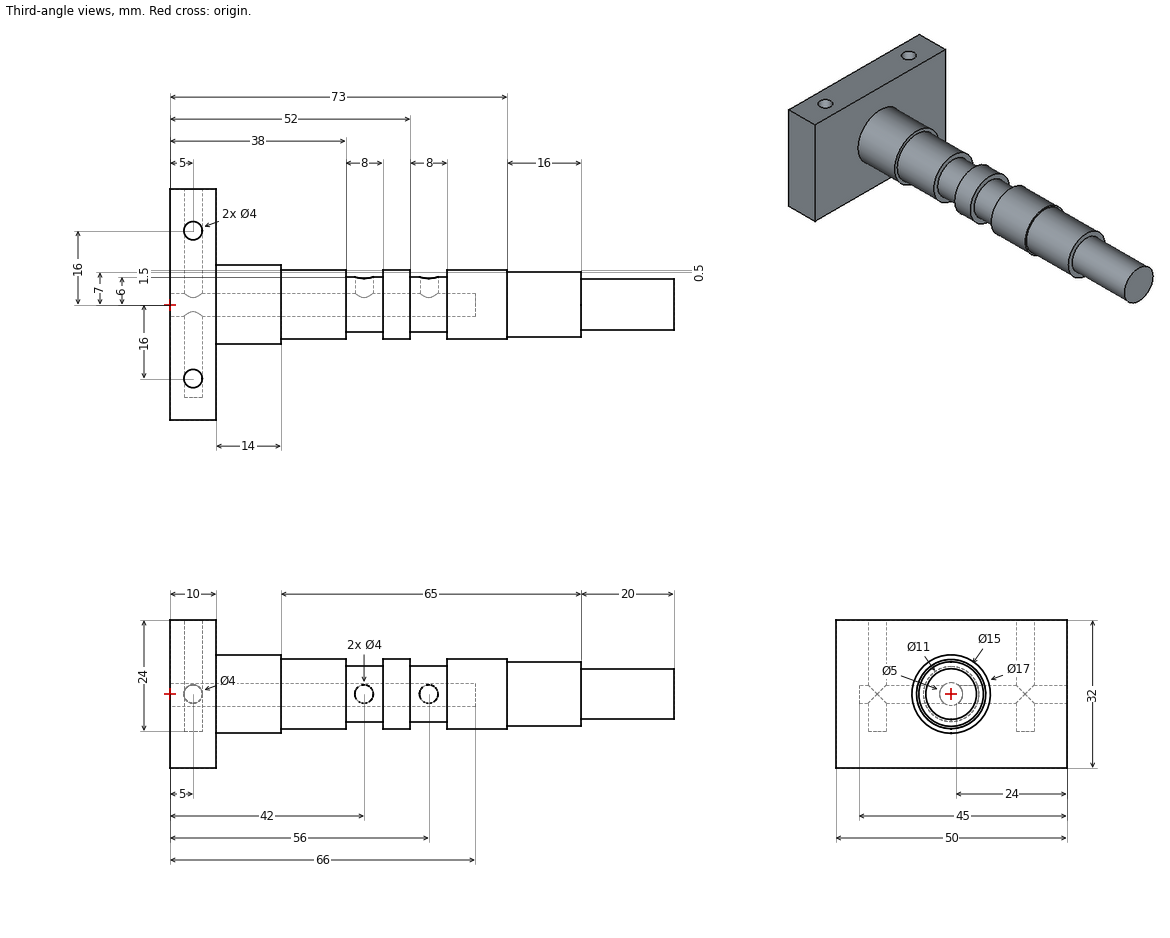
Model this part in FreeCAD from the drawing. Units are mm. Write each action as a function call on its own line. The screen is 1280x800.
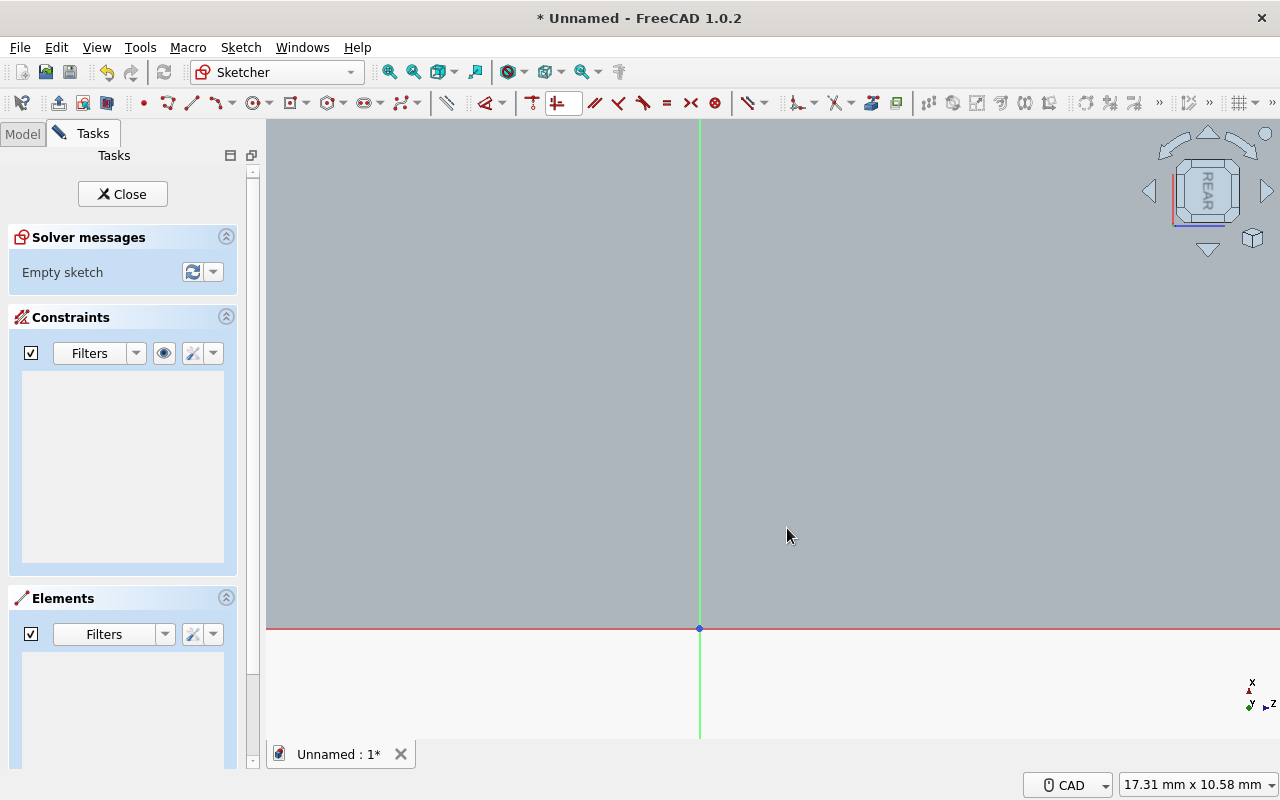
click(254, 104)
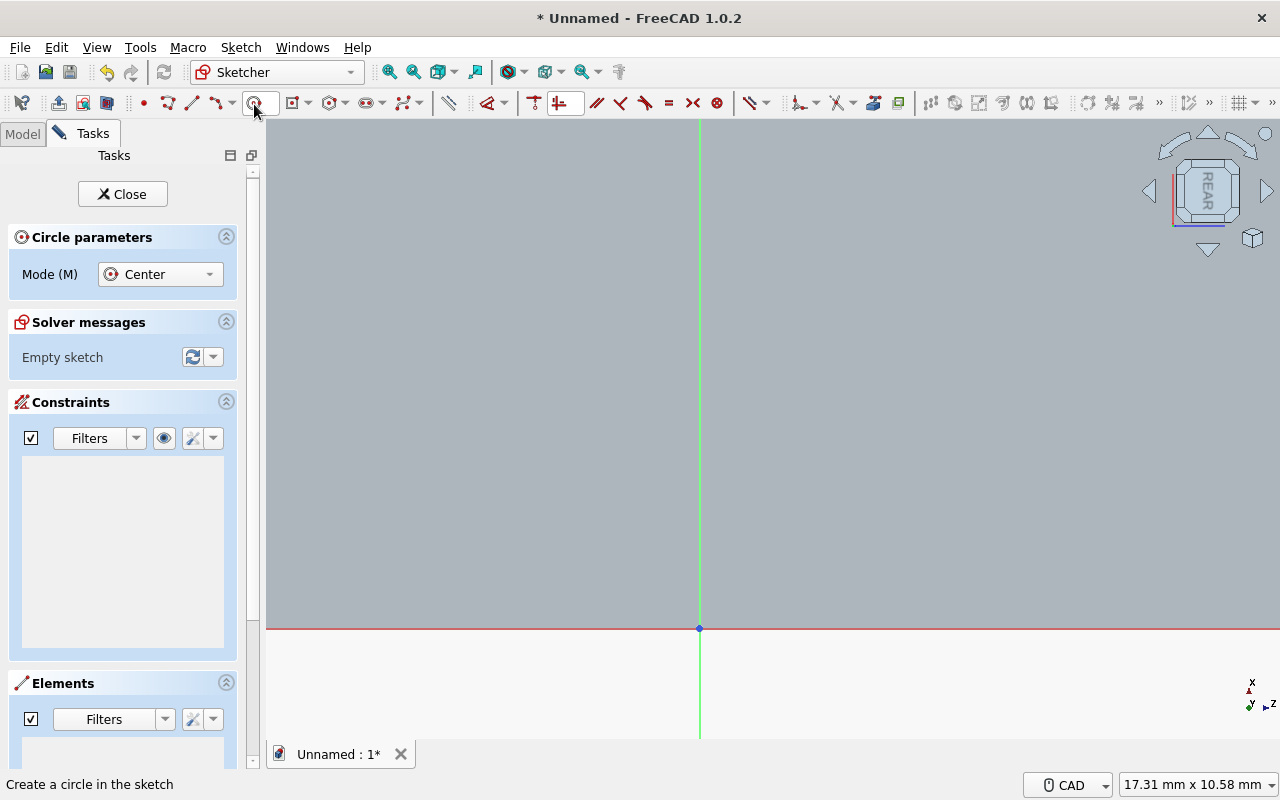
click(700, 336)
move(783, 253)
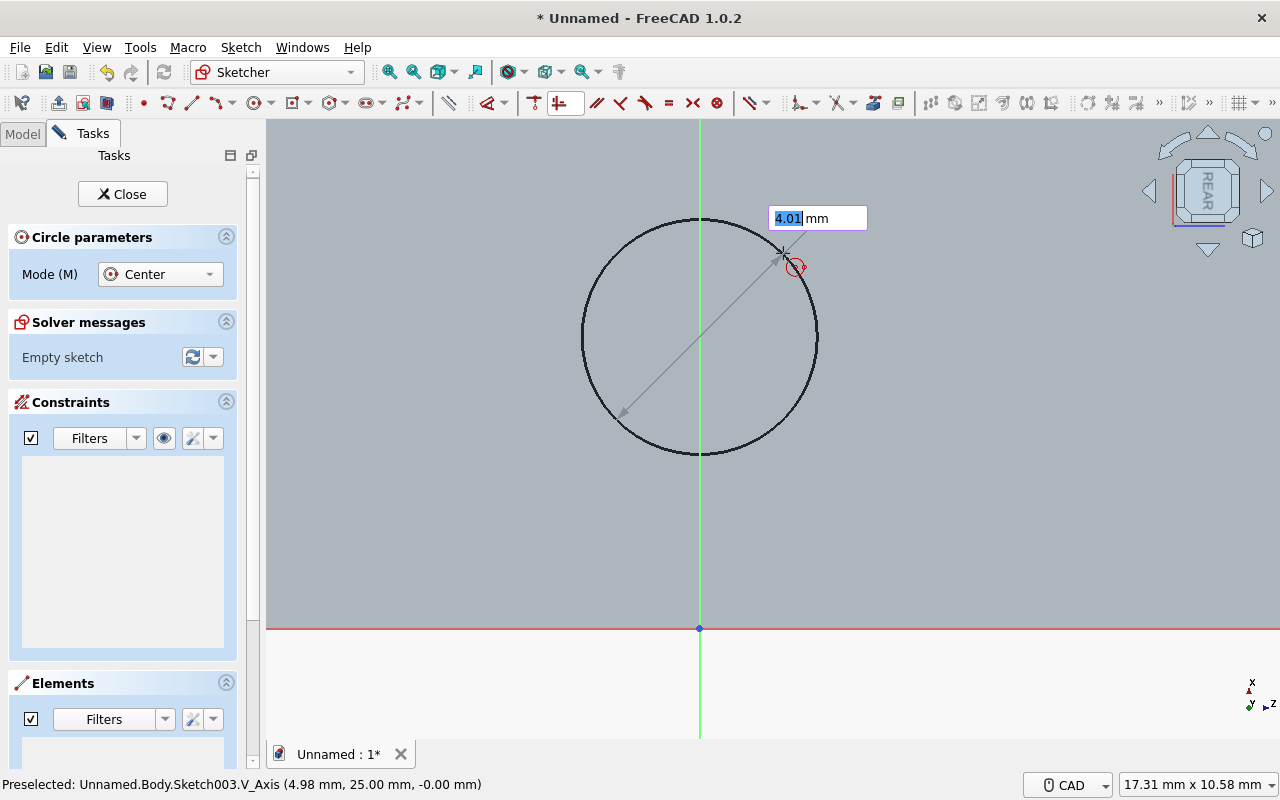
text(4)
key(Return)
key(Escape)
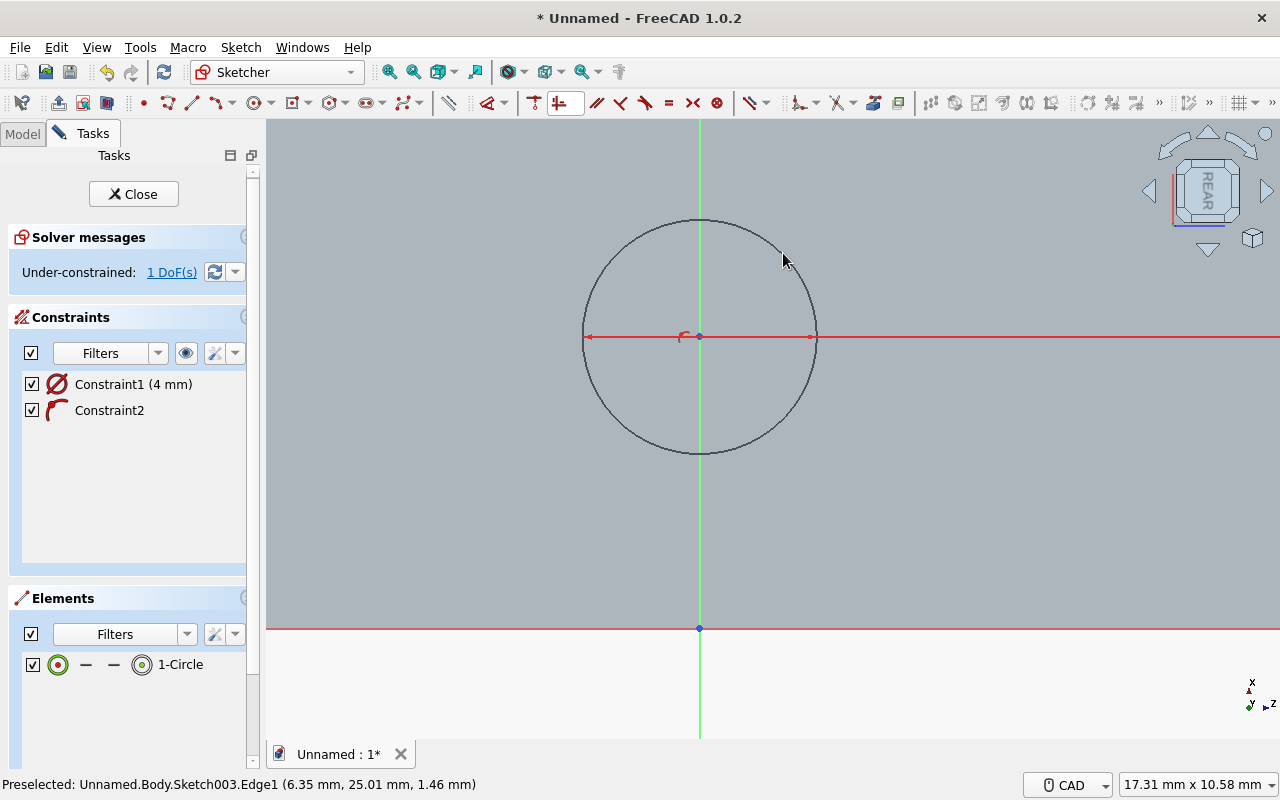
click(488, 104)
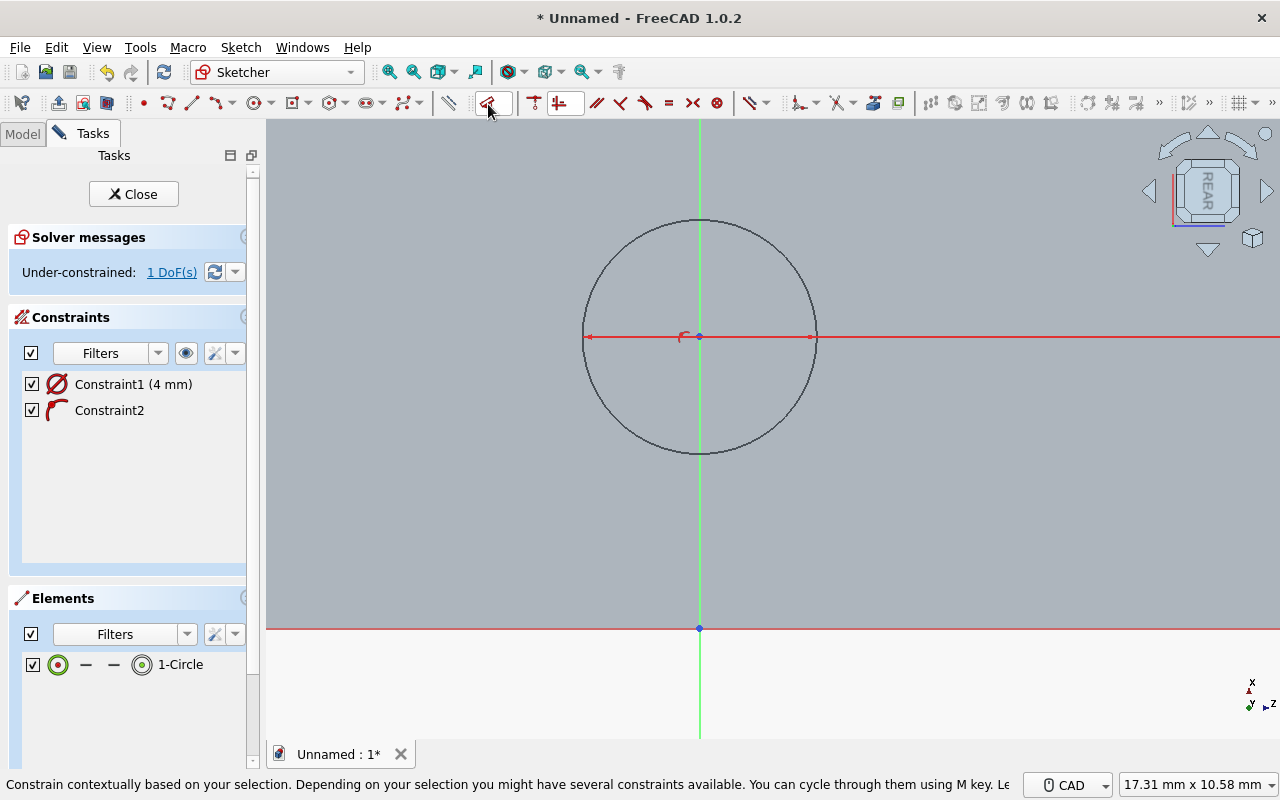
click(700, 337)
click(734, 483)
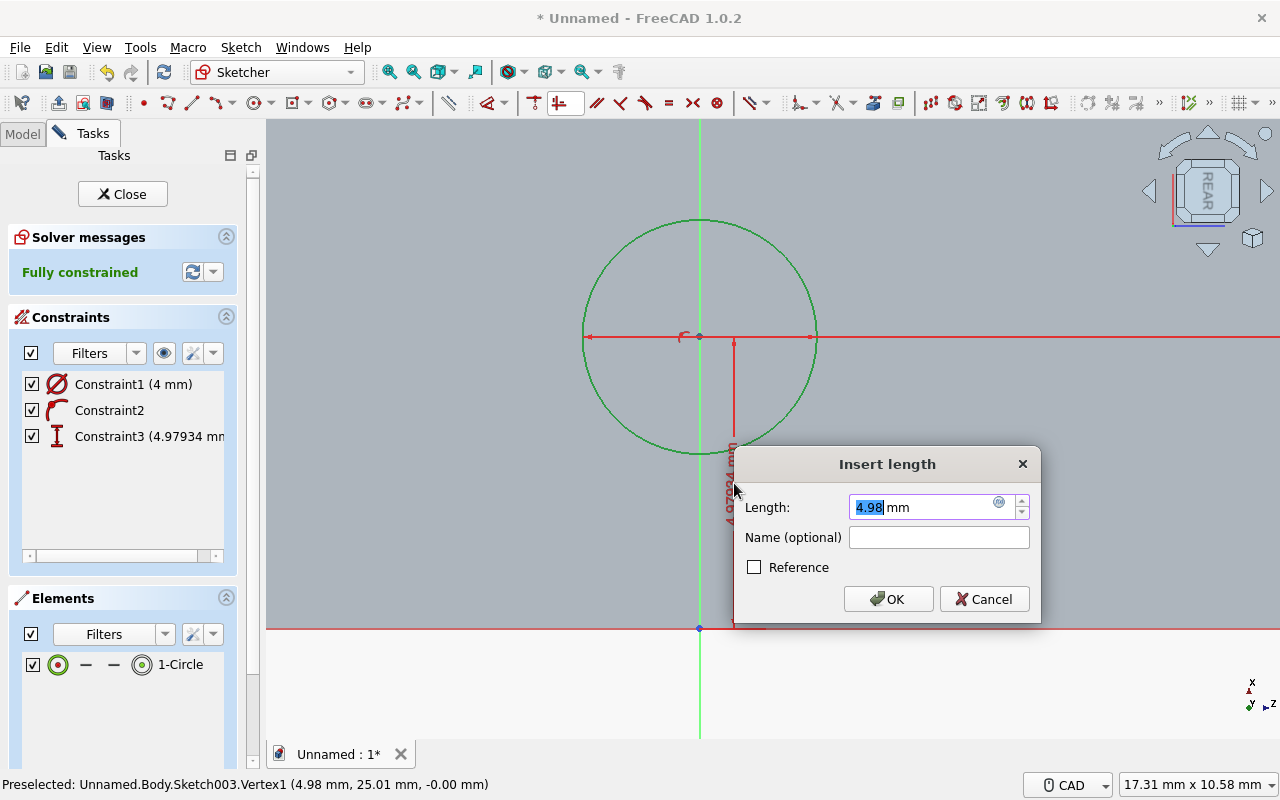
text(5)
key(Return)
key(Escape)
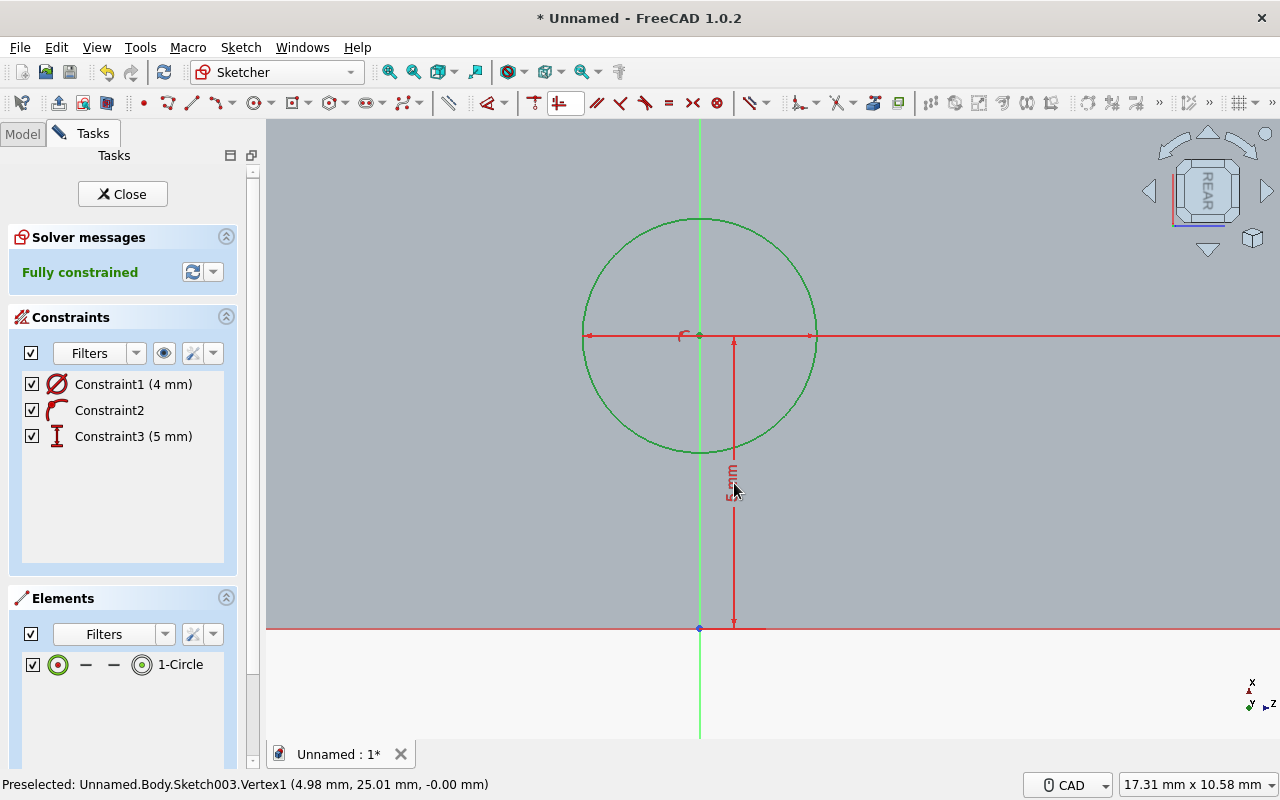
click(123, 194)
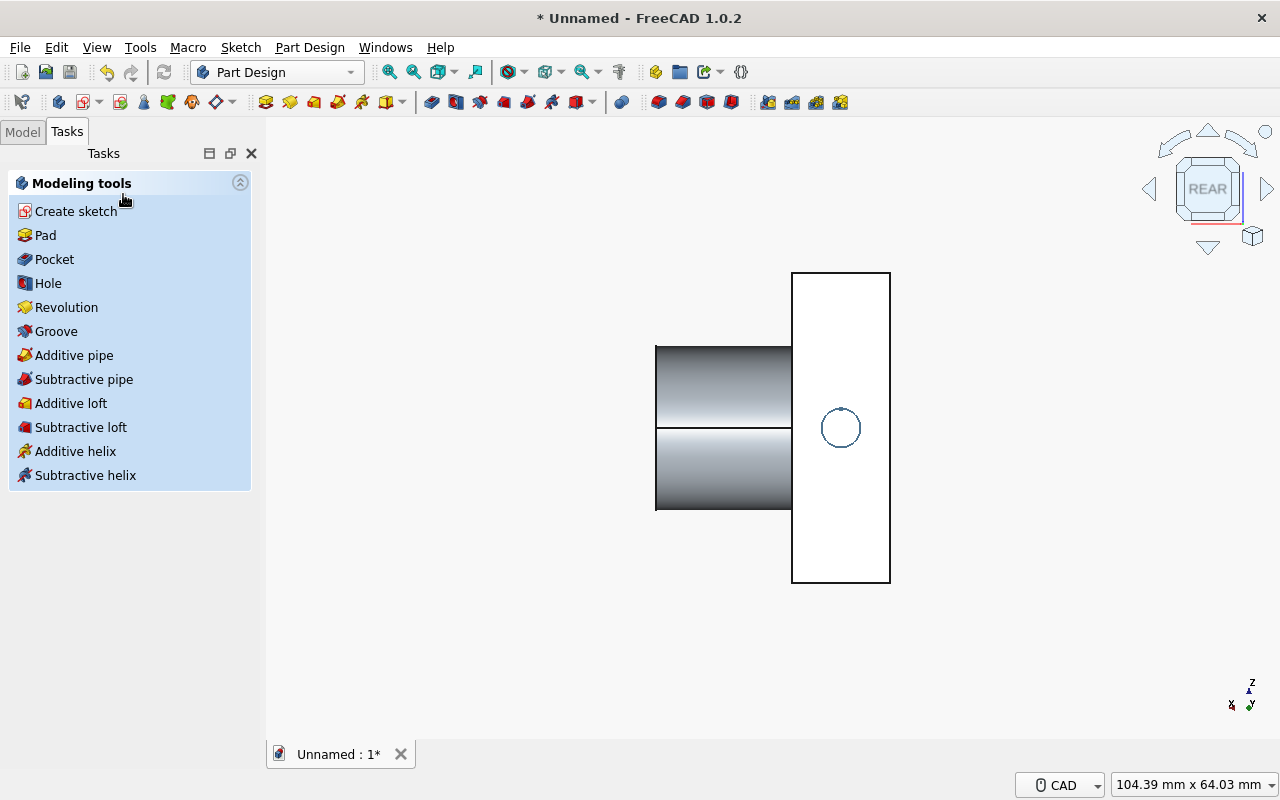
click(432, 102)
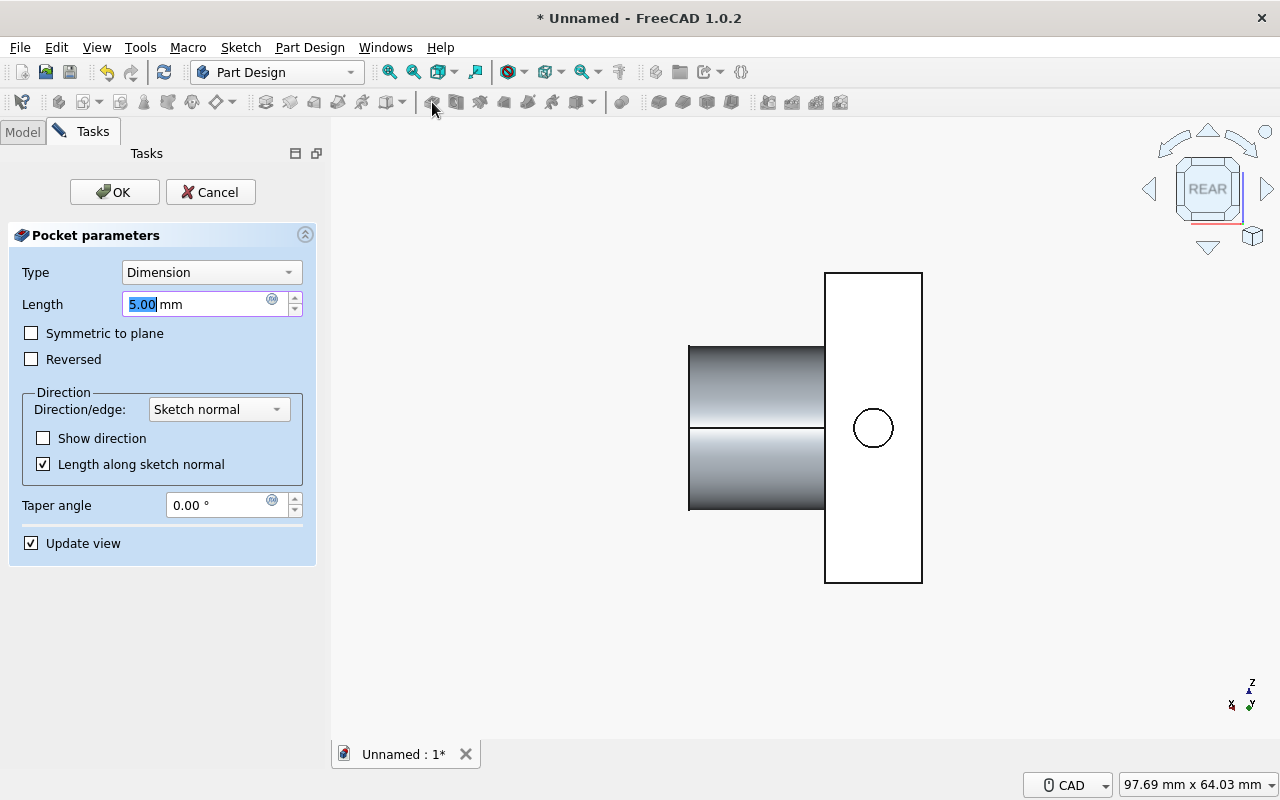
text(45)
key(Tab)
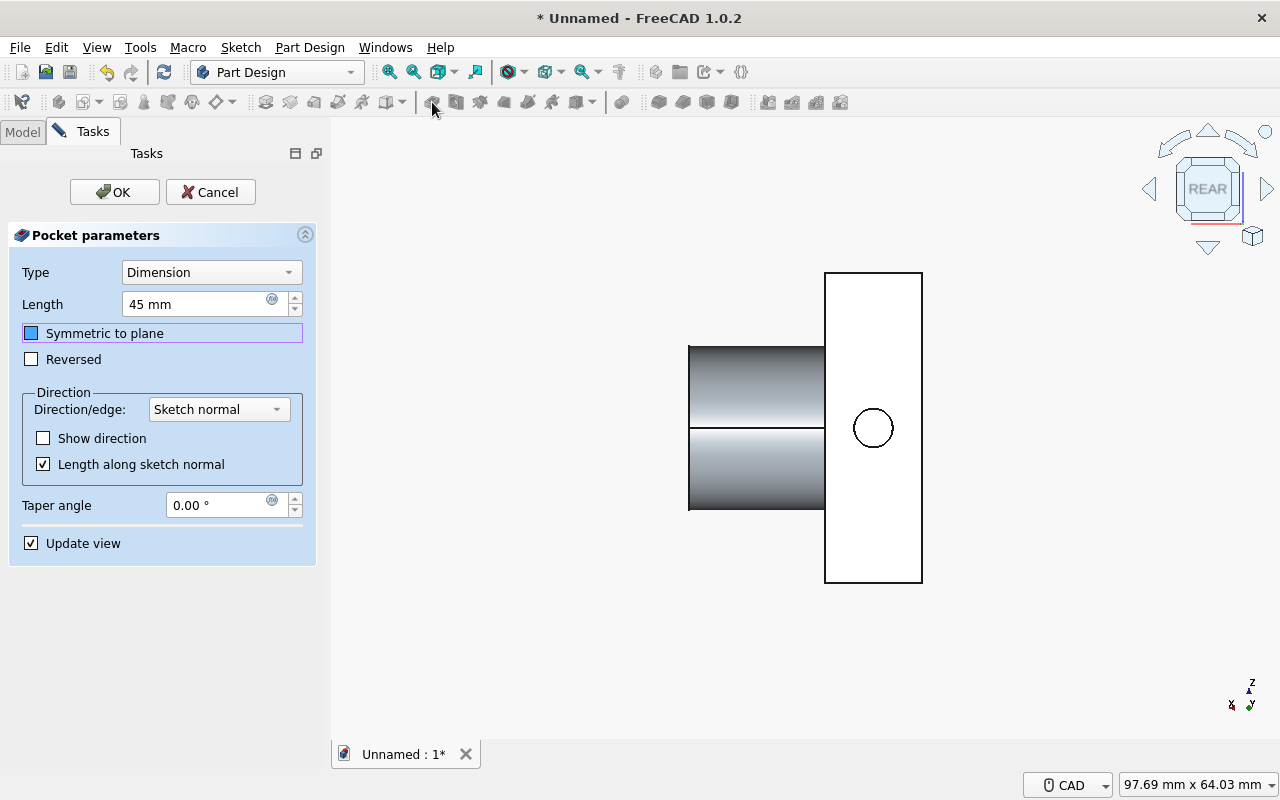
click(115, 192)